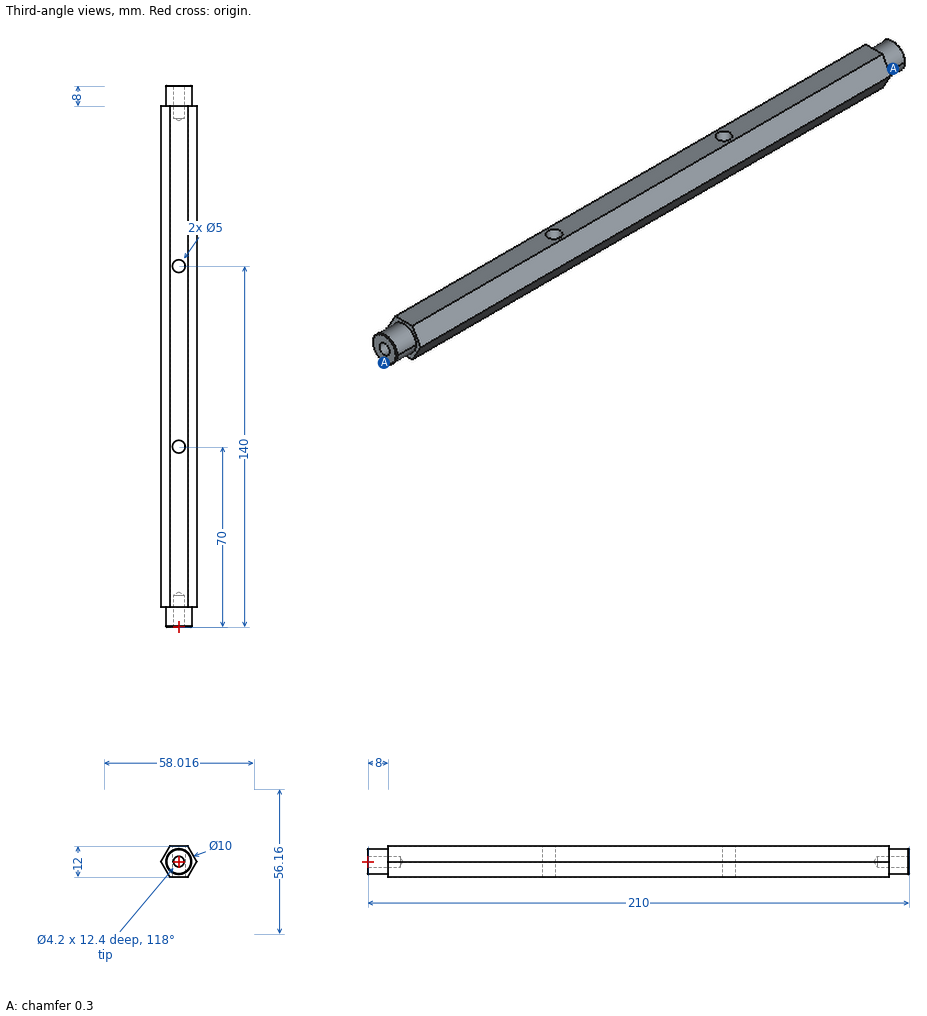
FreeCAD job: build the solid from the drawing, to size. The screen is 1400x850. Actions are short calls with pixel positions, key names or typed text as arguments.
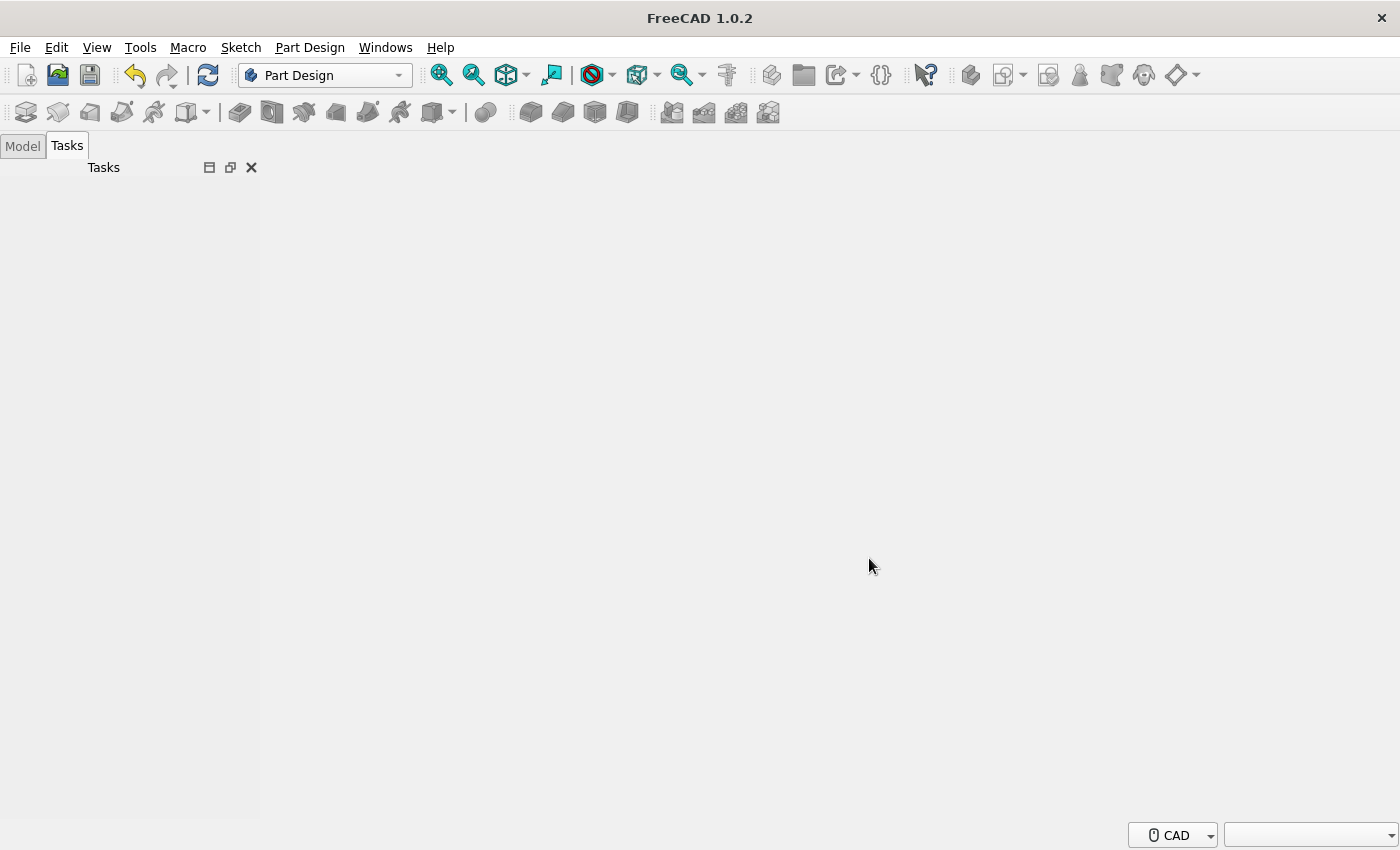
key(ctrl+n)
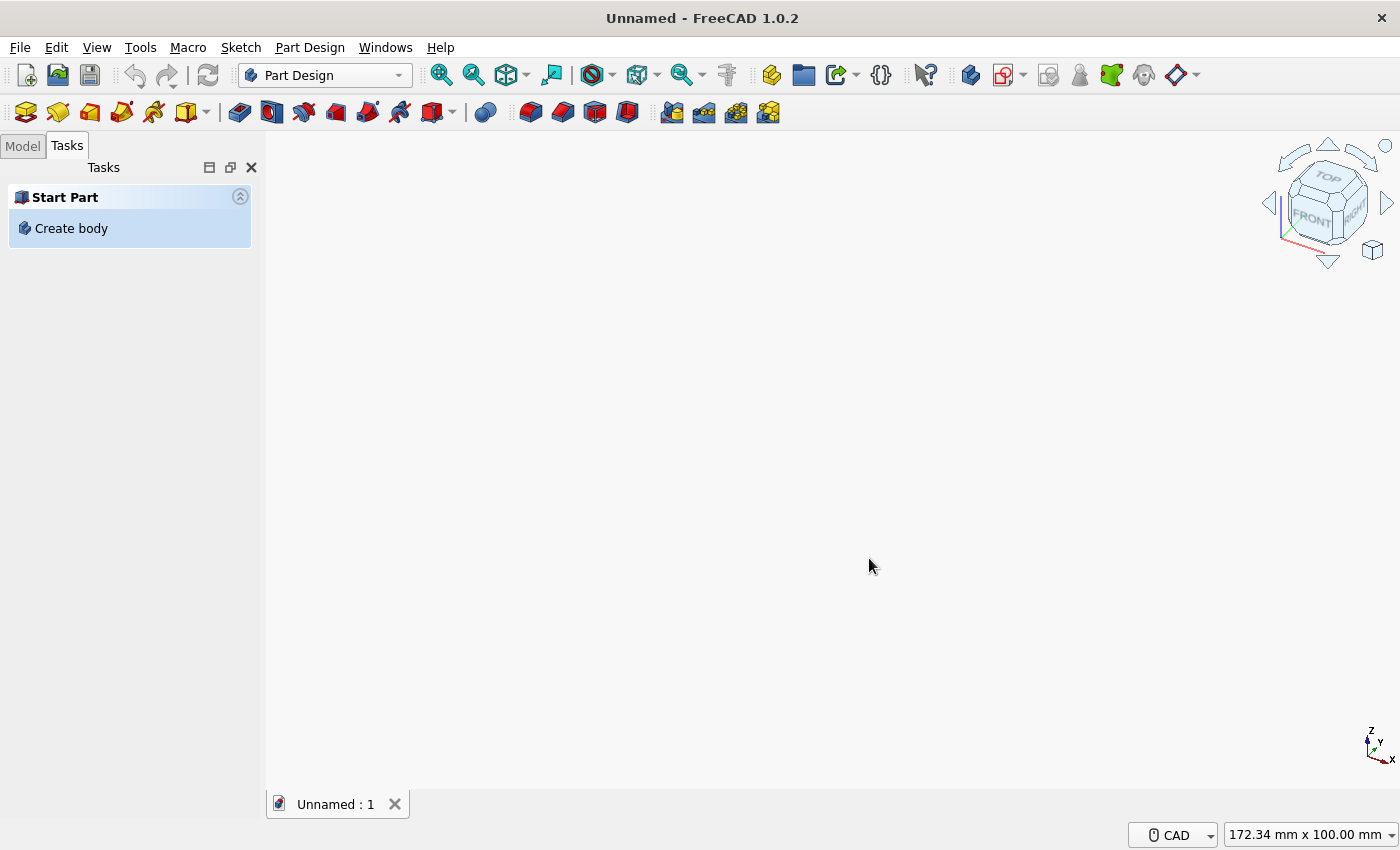
click(1004, 76)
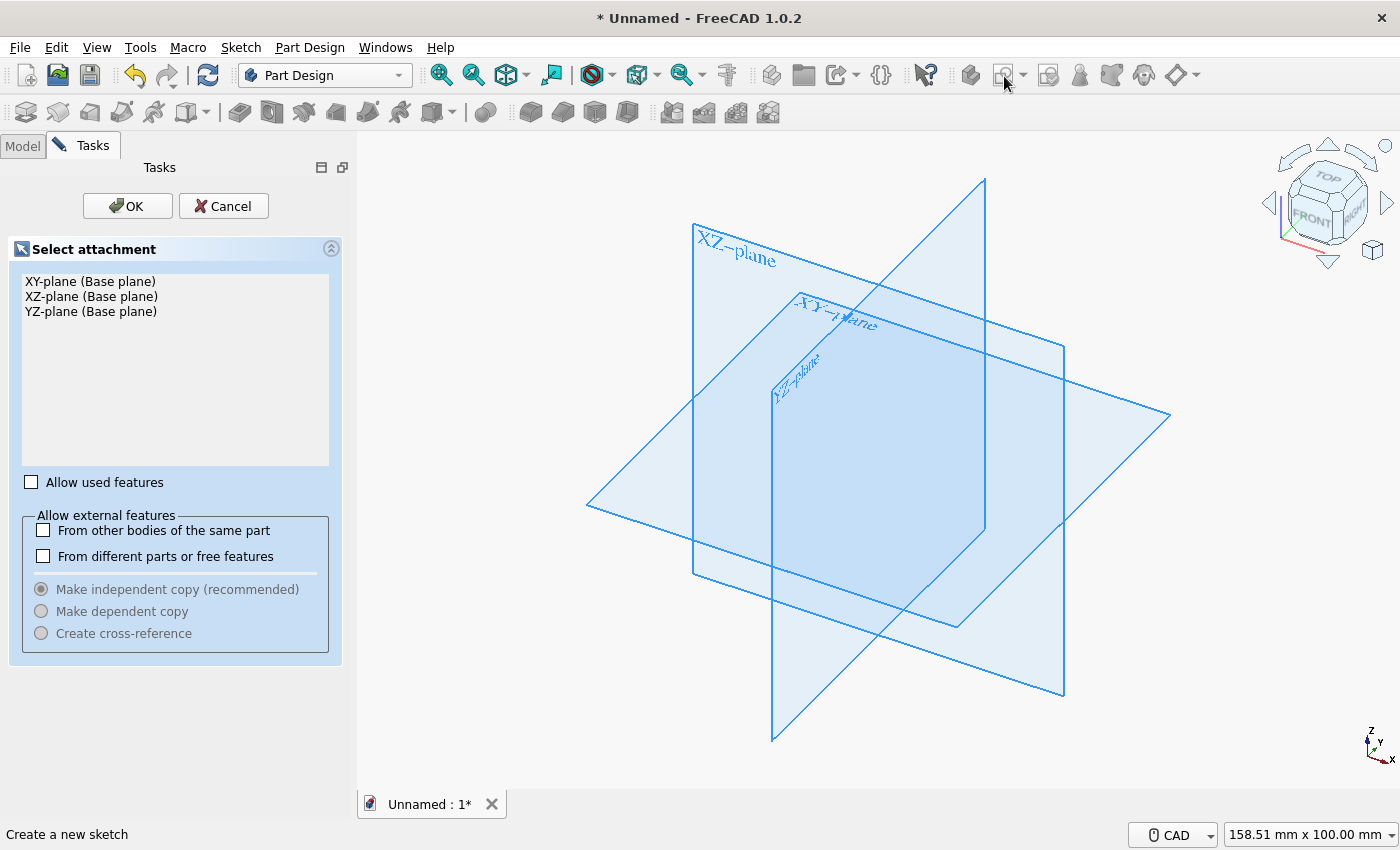
click(82, 296)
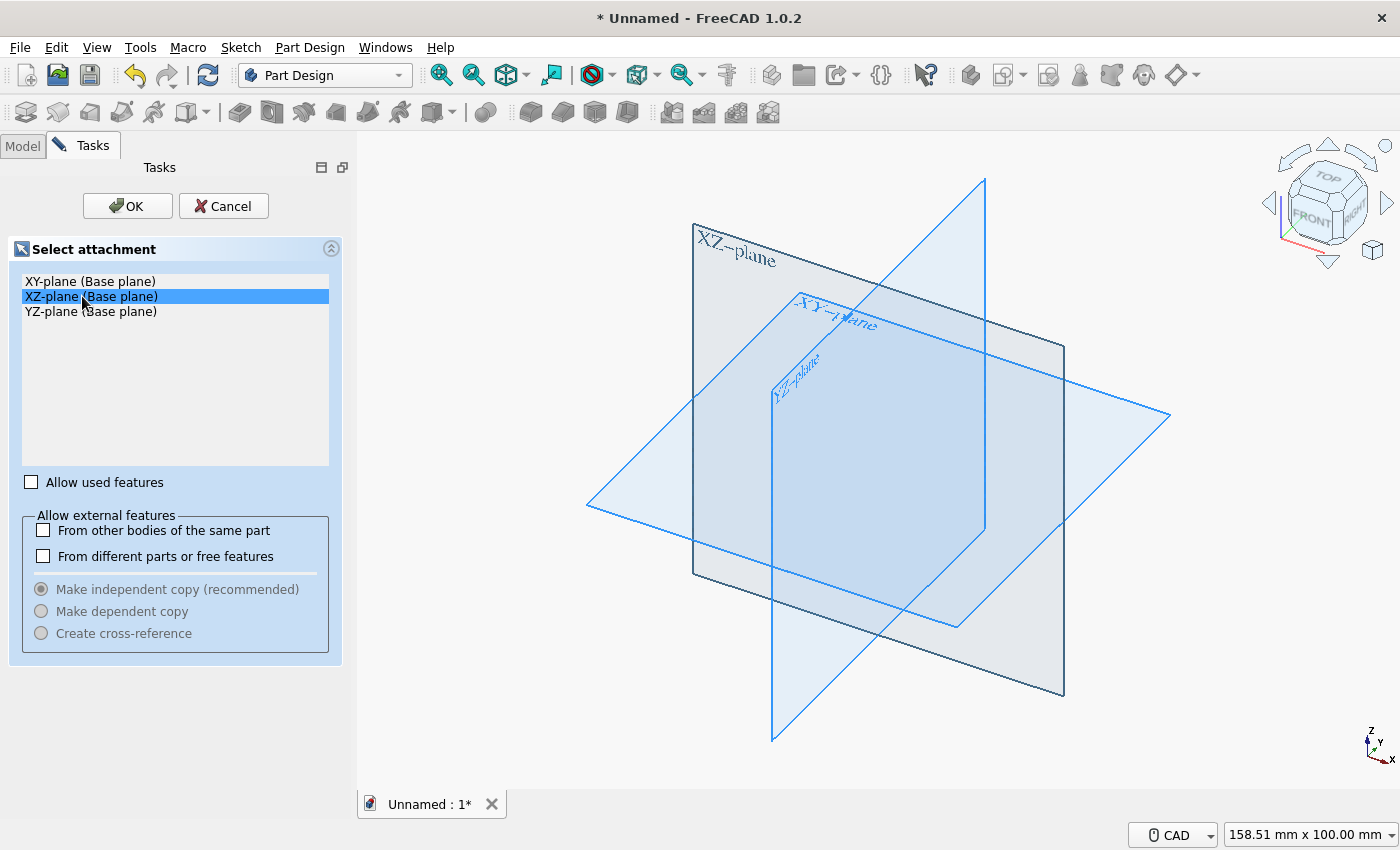
click(128, 206)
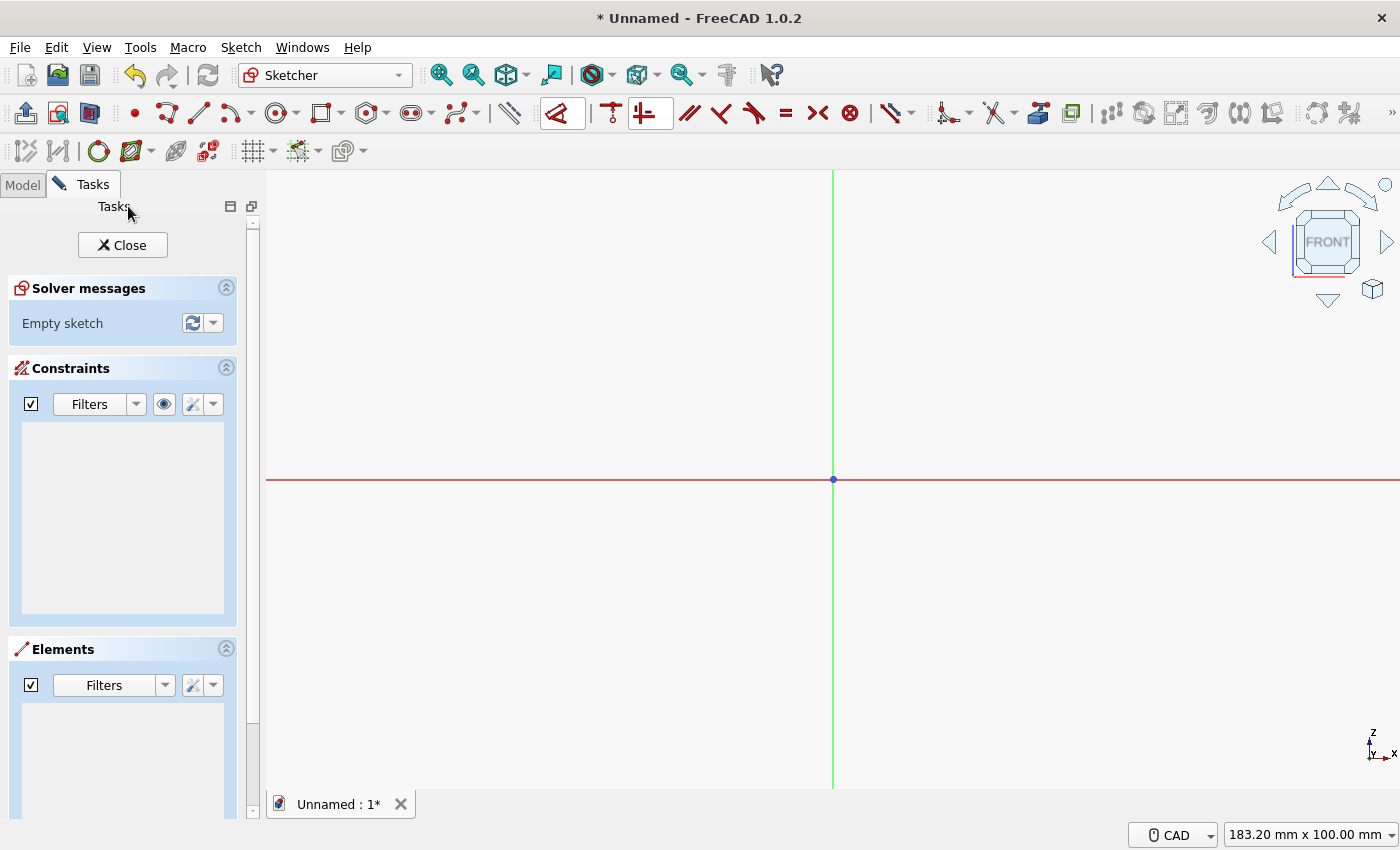
scroll(850, 479, up, 8)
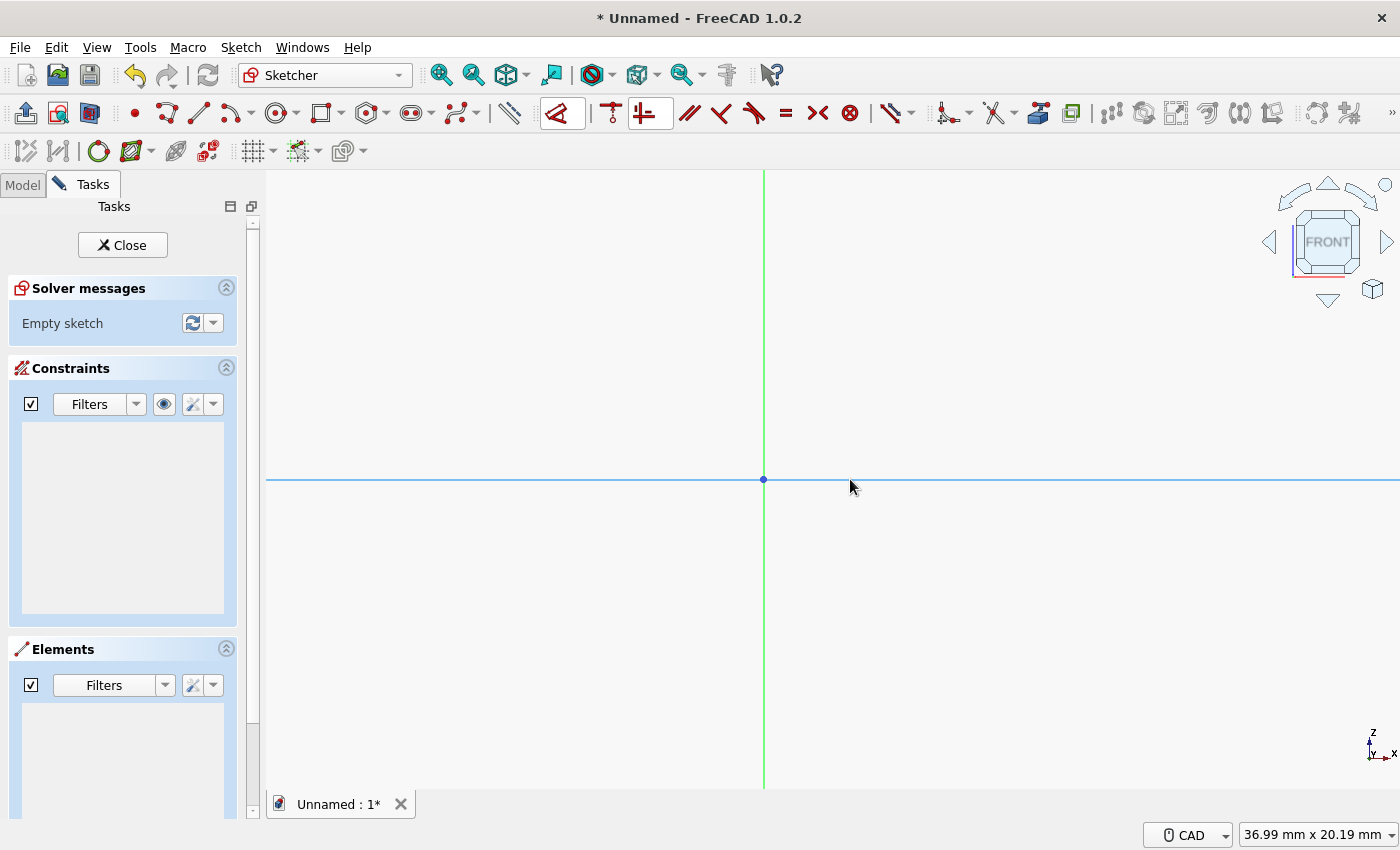
click(366, 114)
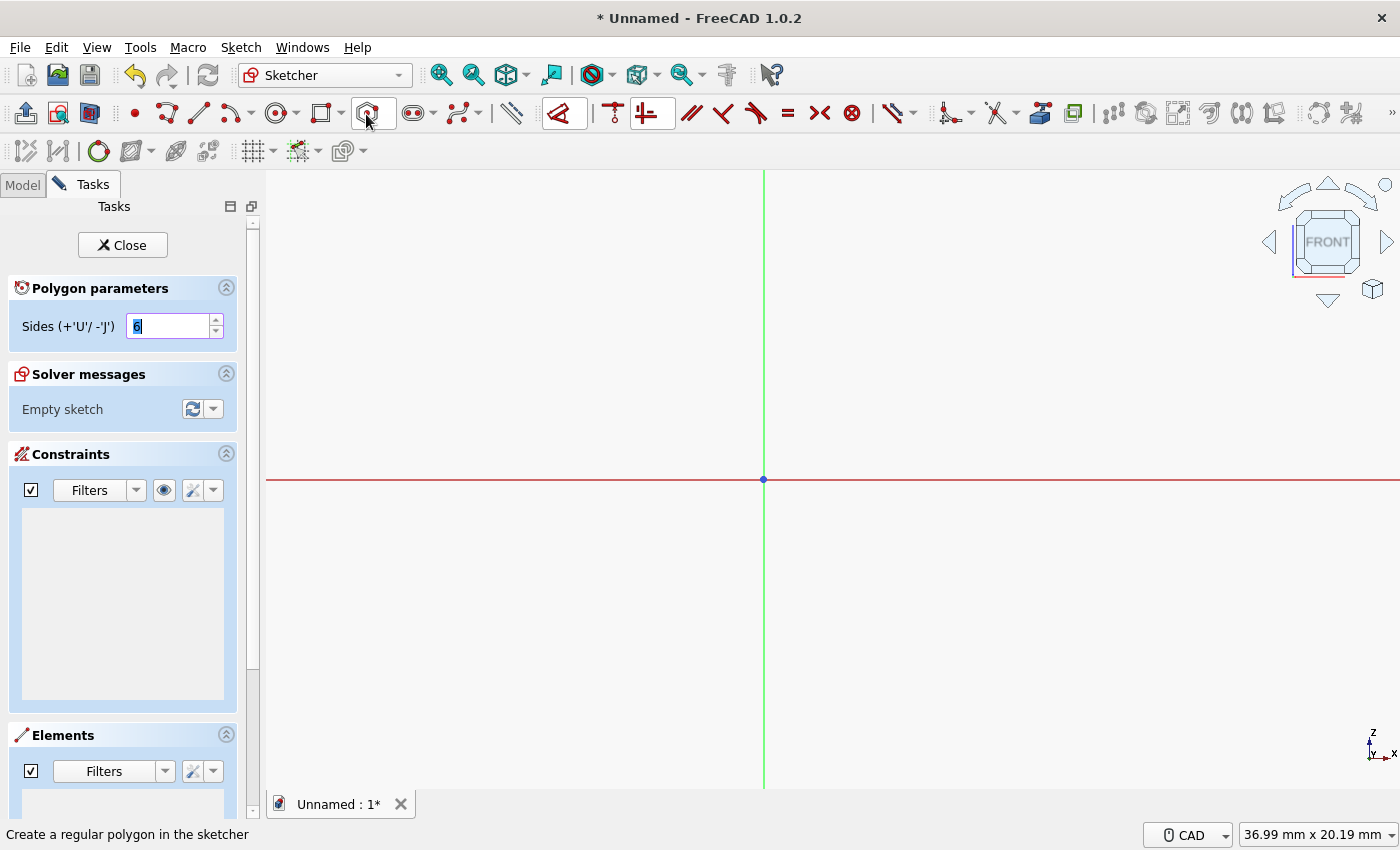
click(764, 480)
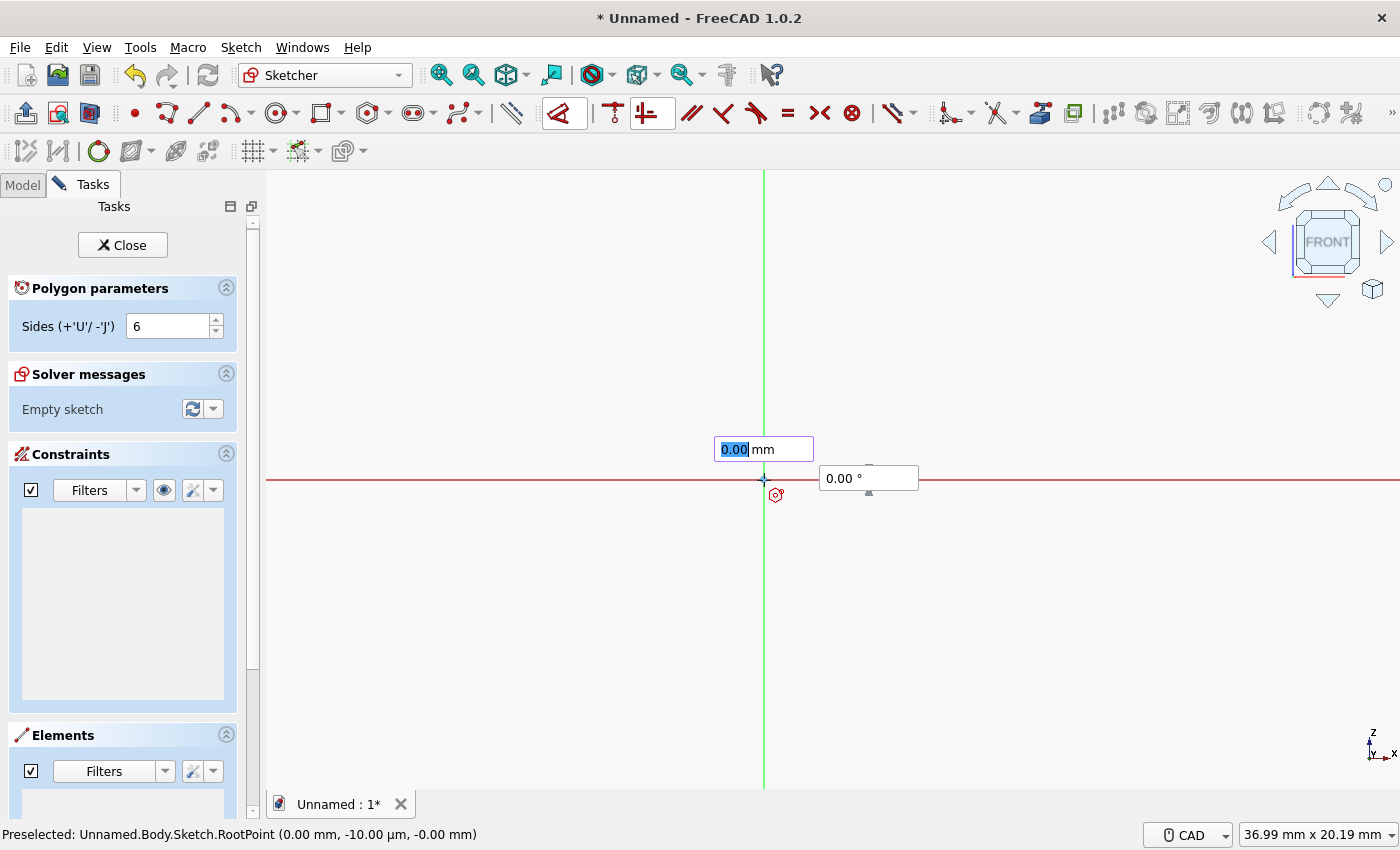
click(976, 480)
right_click(976, 480)